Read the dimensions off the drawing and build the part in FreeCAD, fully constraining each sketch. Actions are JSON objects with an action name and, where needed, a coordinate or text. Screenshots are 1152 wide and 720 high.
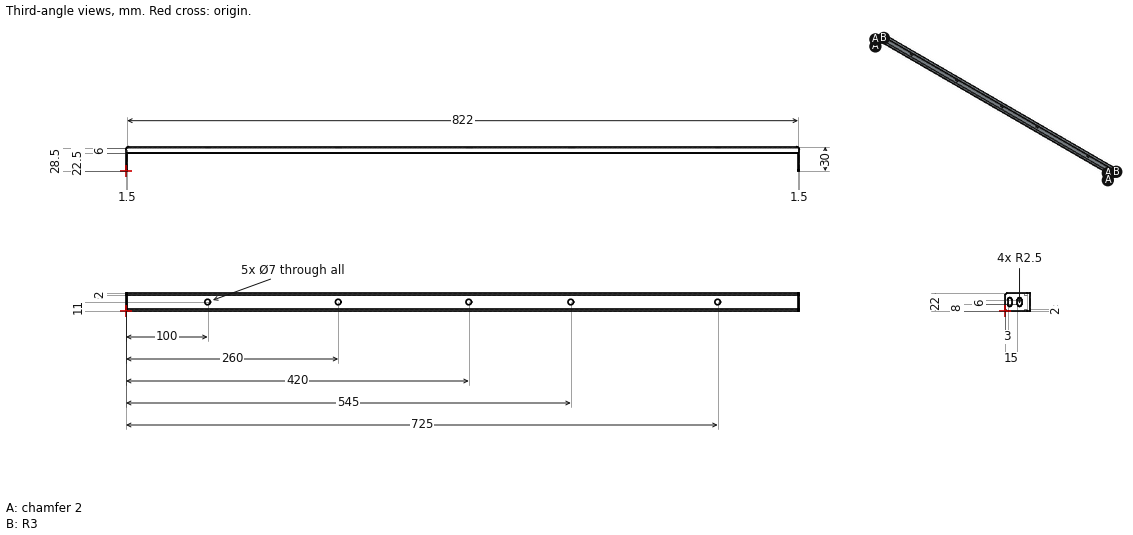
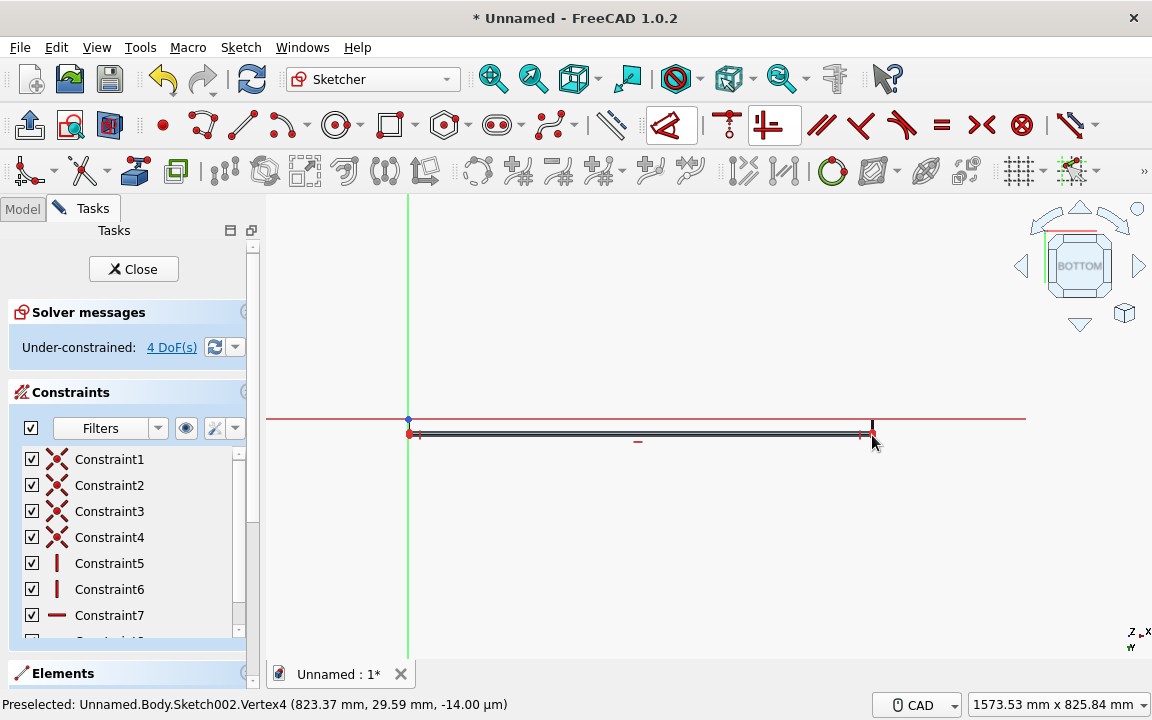
{"action": "scroll", "coordinate": [409, 434], "scroll_direction": "up", "scroll_amount": 13}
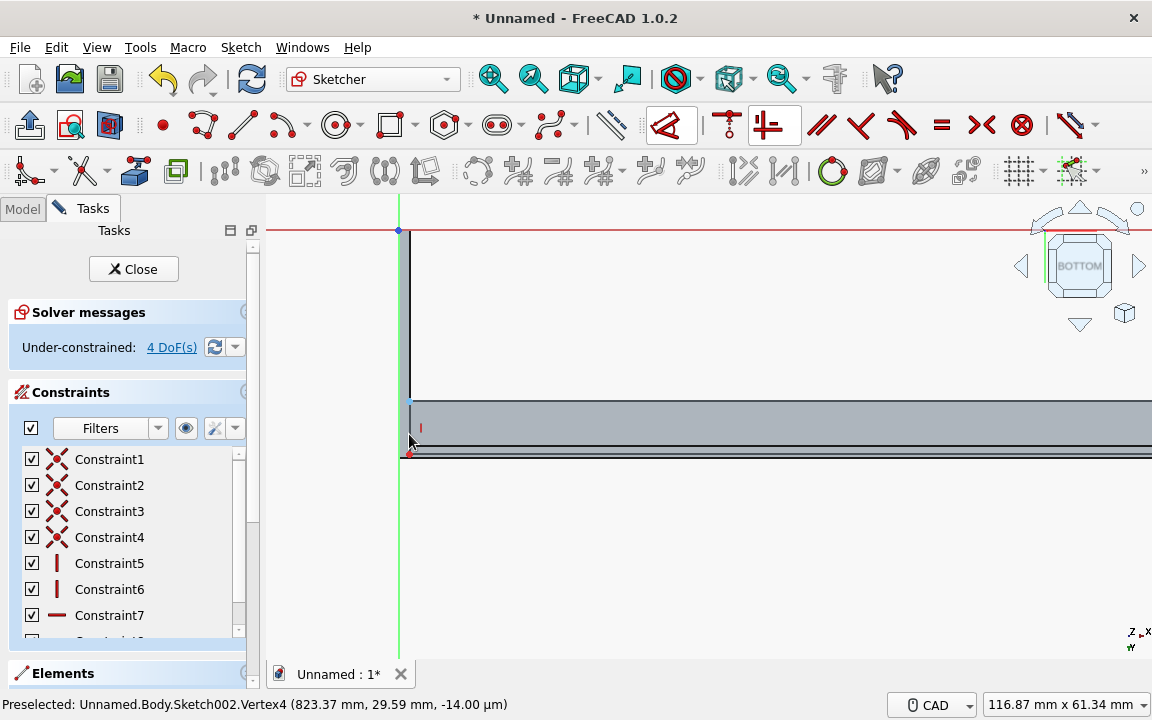
{"action": "left_click", "coordinate": [410, 428]}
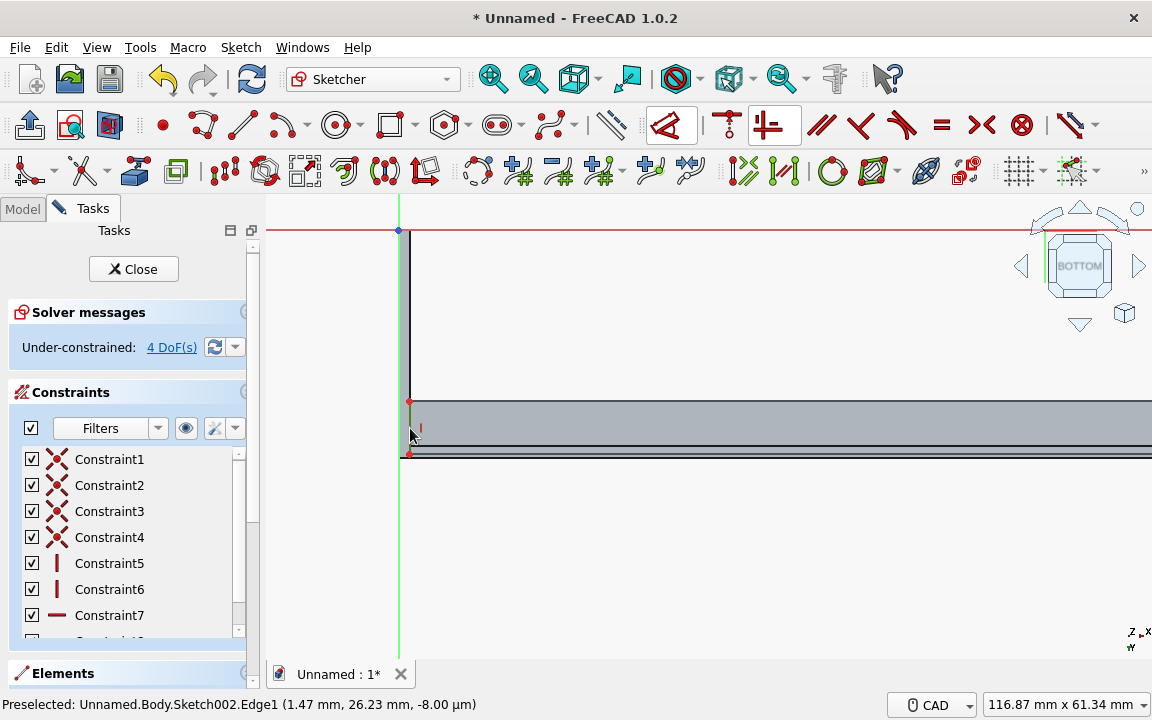
{"action": "left_click", "coordinate": [692, 126]}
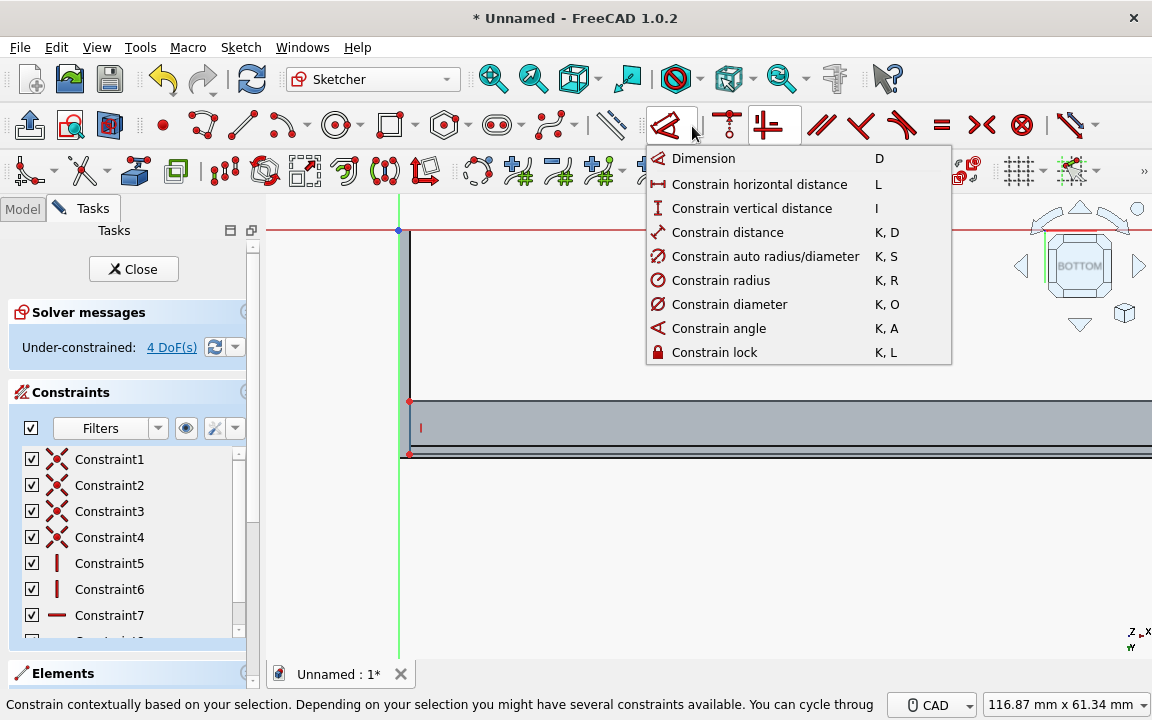
{"action": "left_click", "coordinate": [799, 208]}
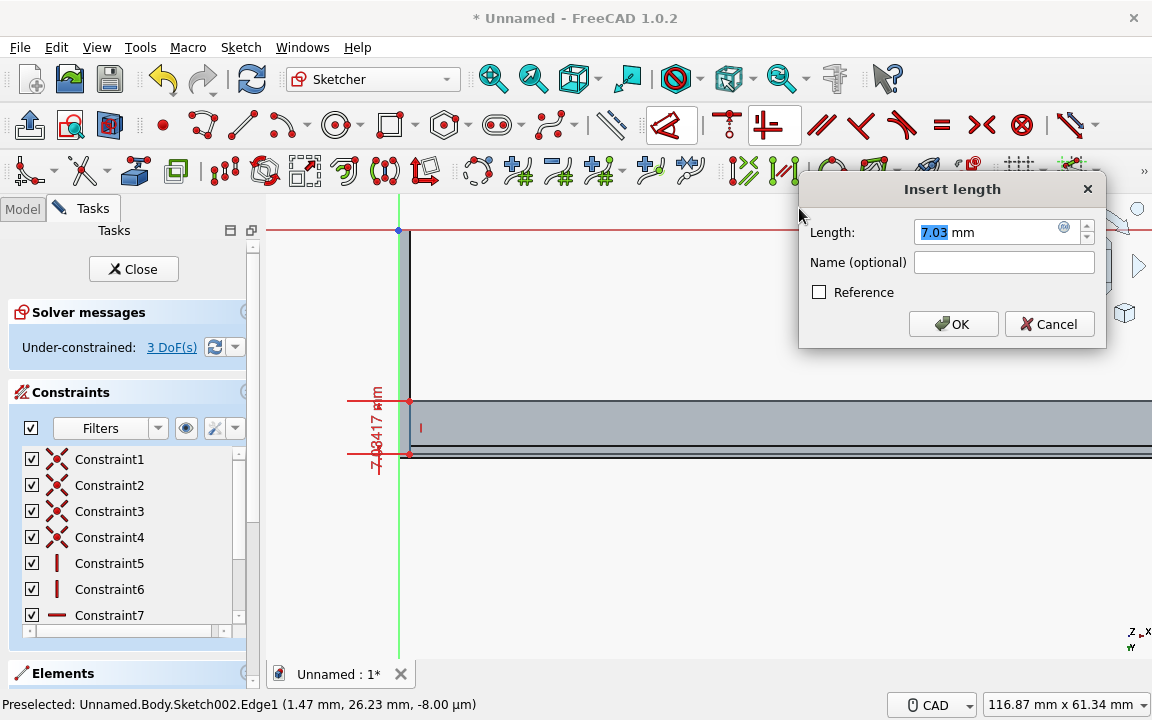
{"action": "type", "text": "6"}
{"action": "key", "text": "Return"}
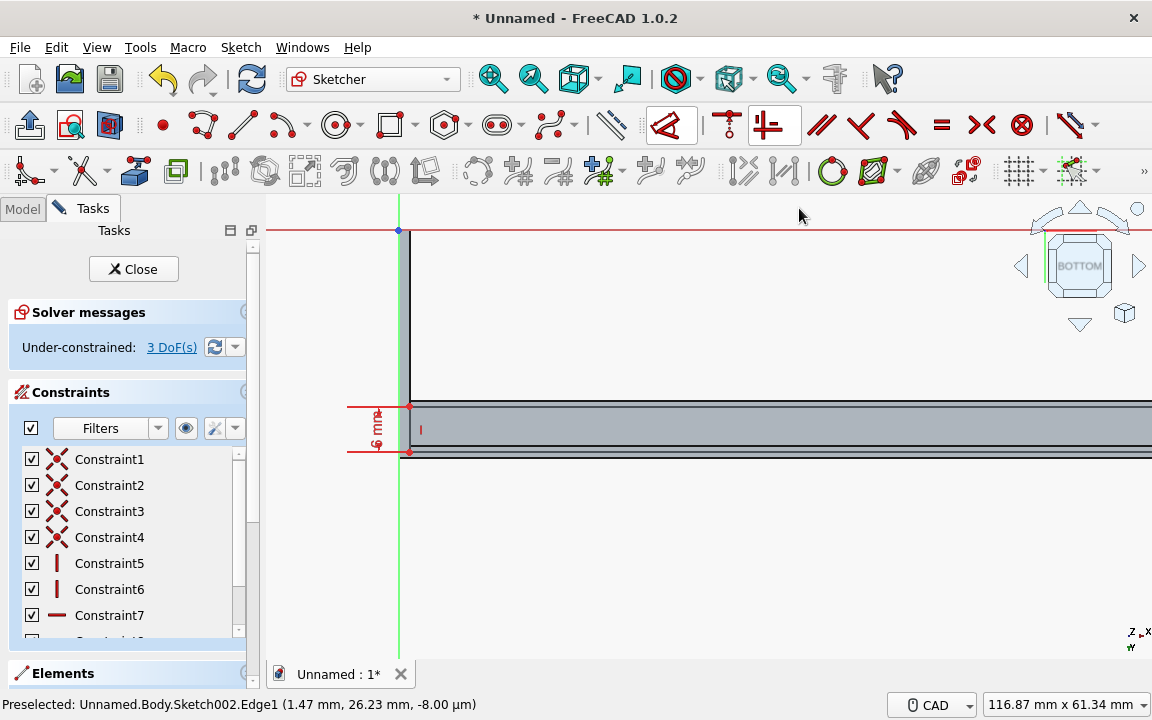
{"action": "scroll", "coordinate": [409, 434], "scroll_direction": "down", "scroll_amount": 13}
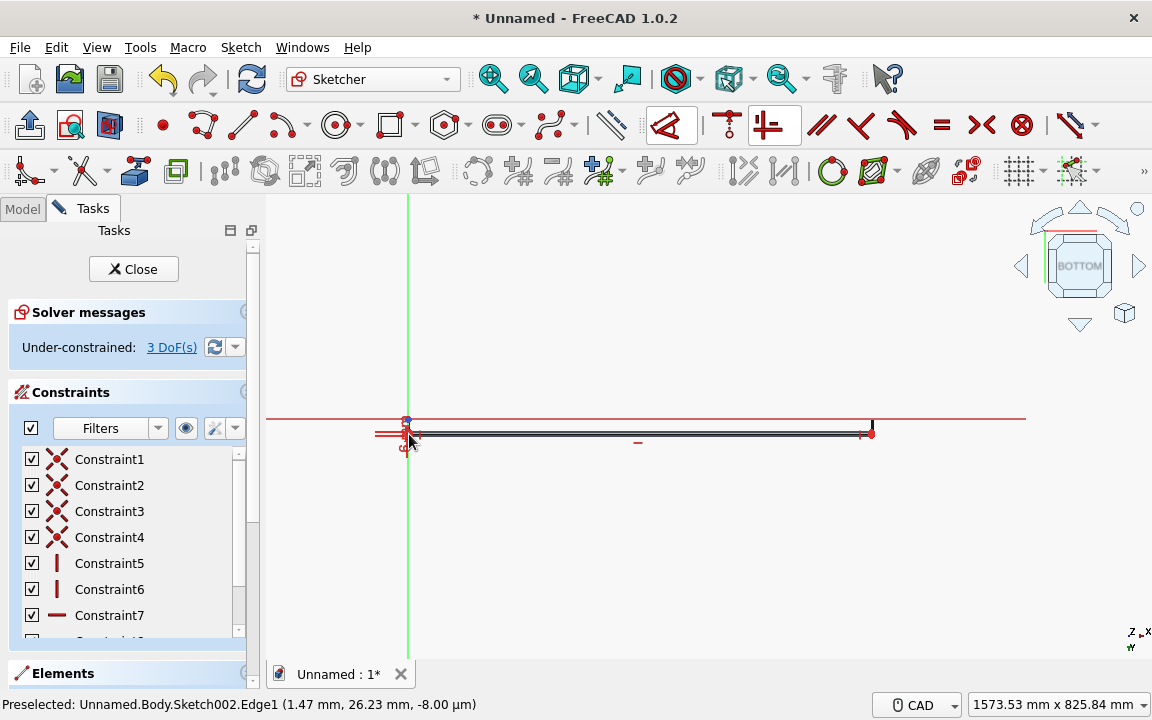
{"action": "scroll", "coordinate": [548, 436], "scroll_direction": "up", "scroll_amount": 8}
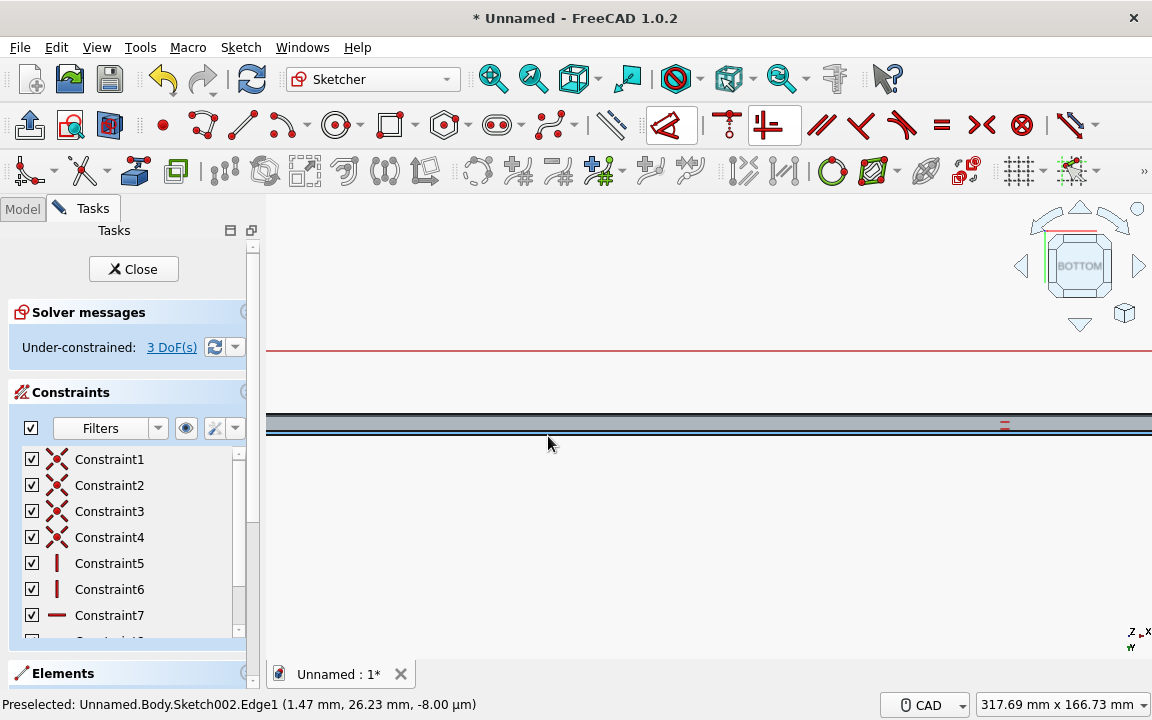
{"action": "left_click", "coordinate": [547, 433]}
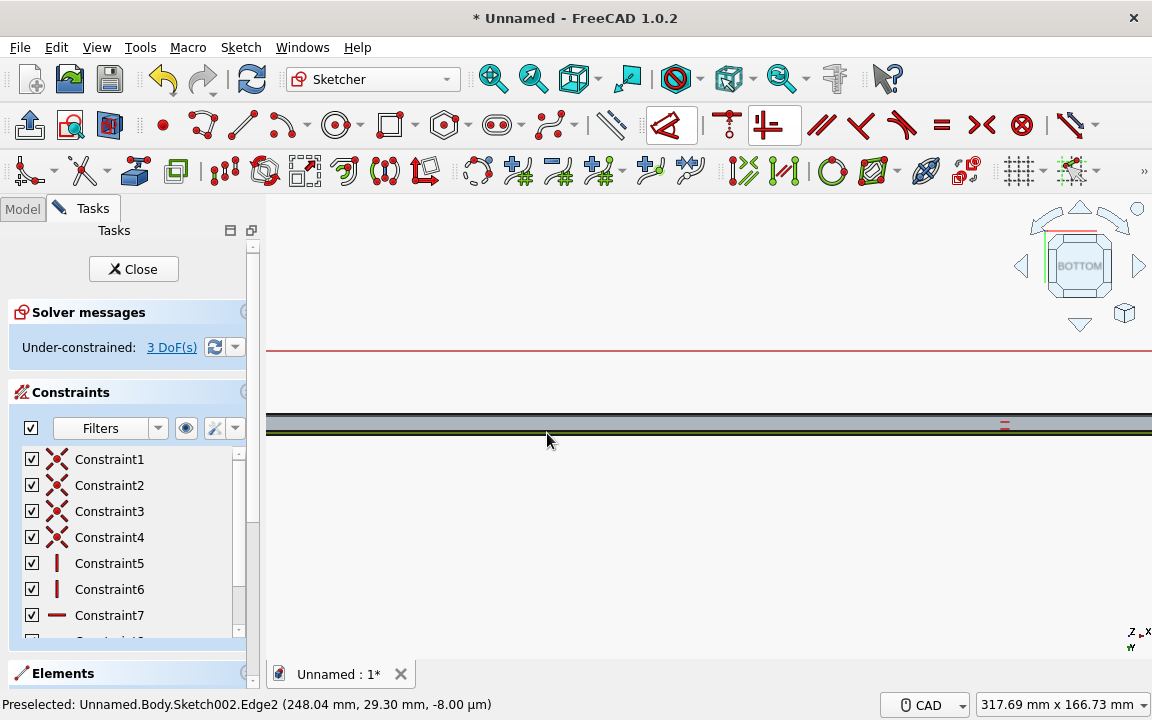
{"action": "key", "text": "l"}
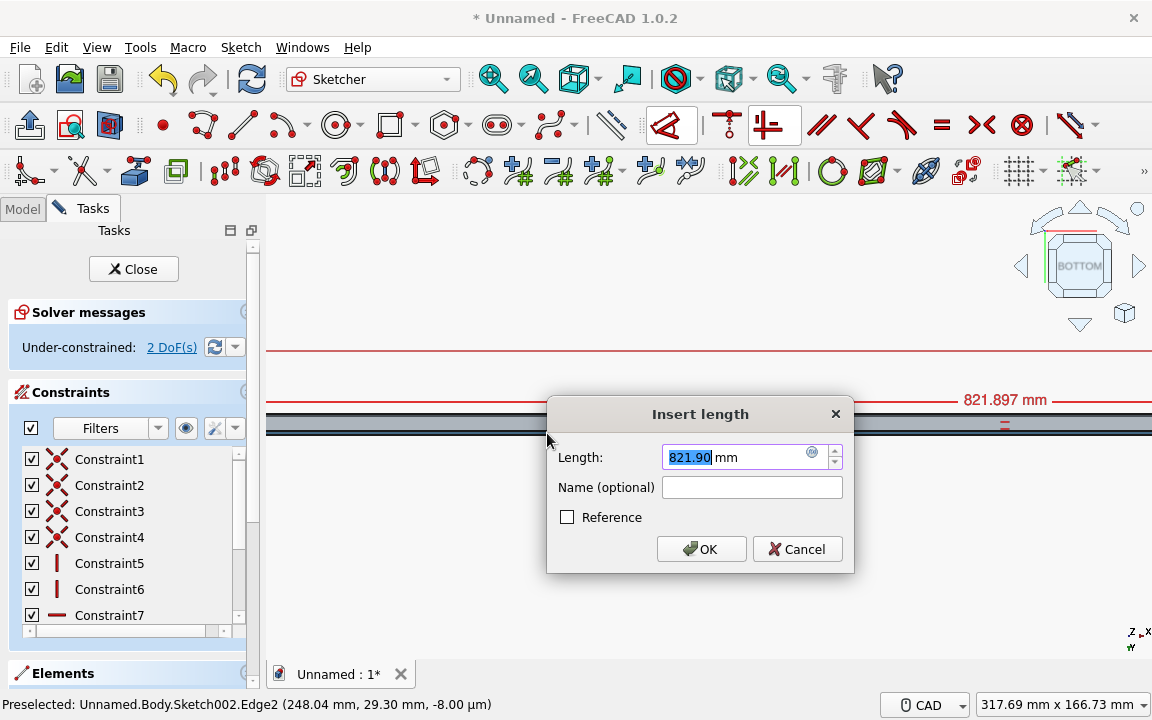
{"action": "type", "text": "822"}
{"action": "key", "text": "Return"}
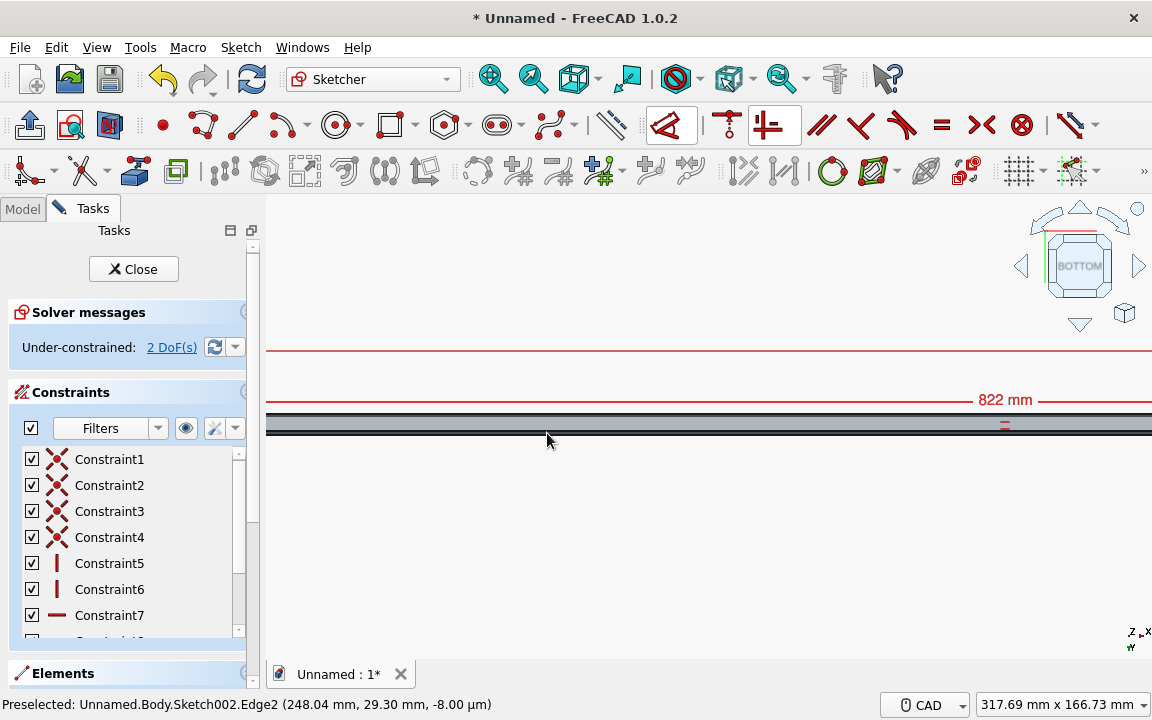
{"action": "scroll", "coordinate": [549, 435], "scroll_direction": "down", "scroll_amount": 8}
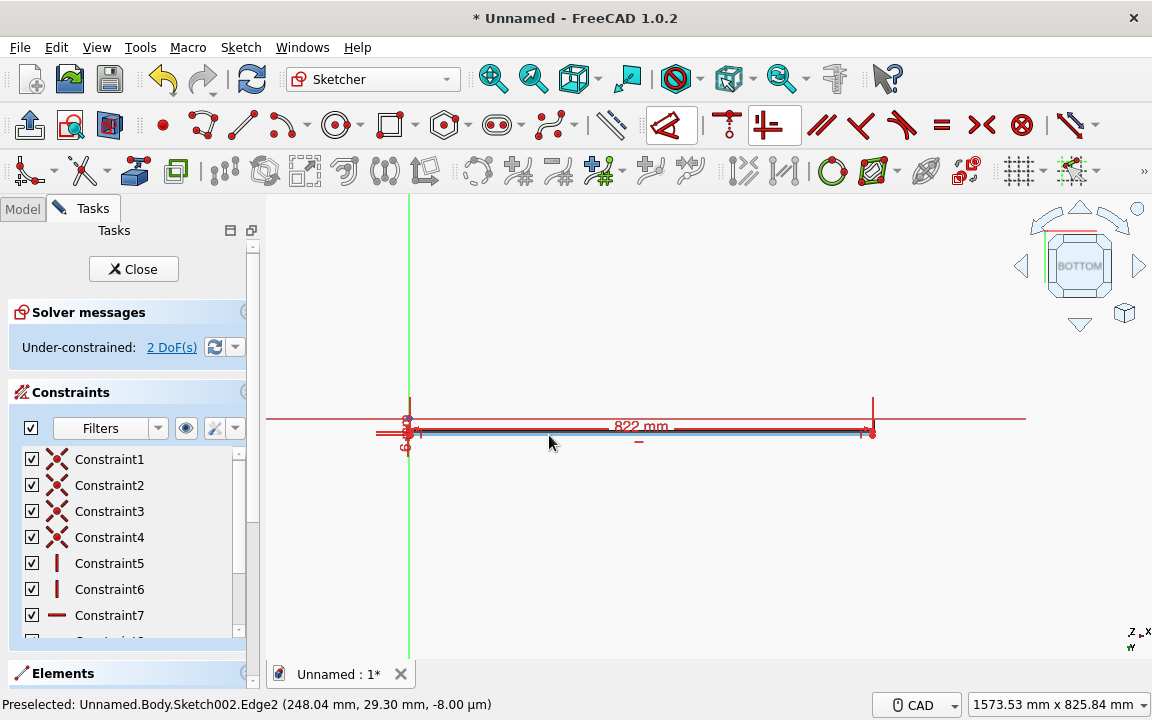
{"action": "scroll", "coordinate": [410, 432], "scroll_direction": "up", "scroll_amount": 20}